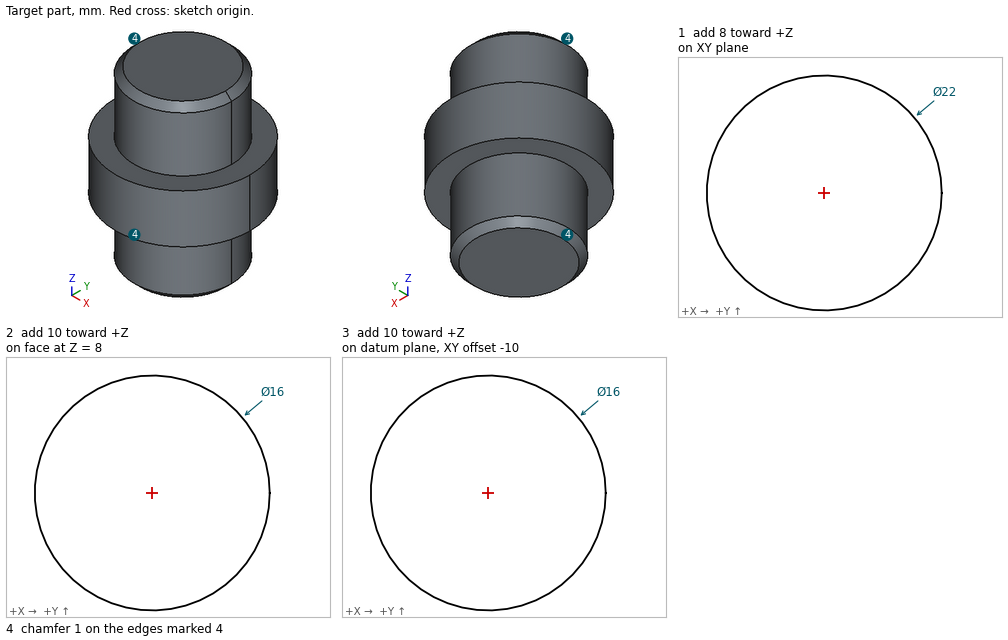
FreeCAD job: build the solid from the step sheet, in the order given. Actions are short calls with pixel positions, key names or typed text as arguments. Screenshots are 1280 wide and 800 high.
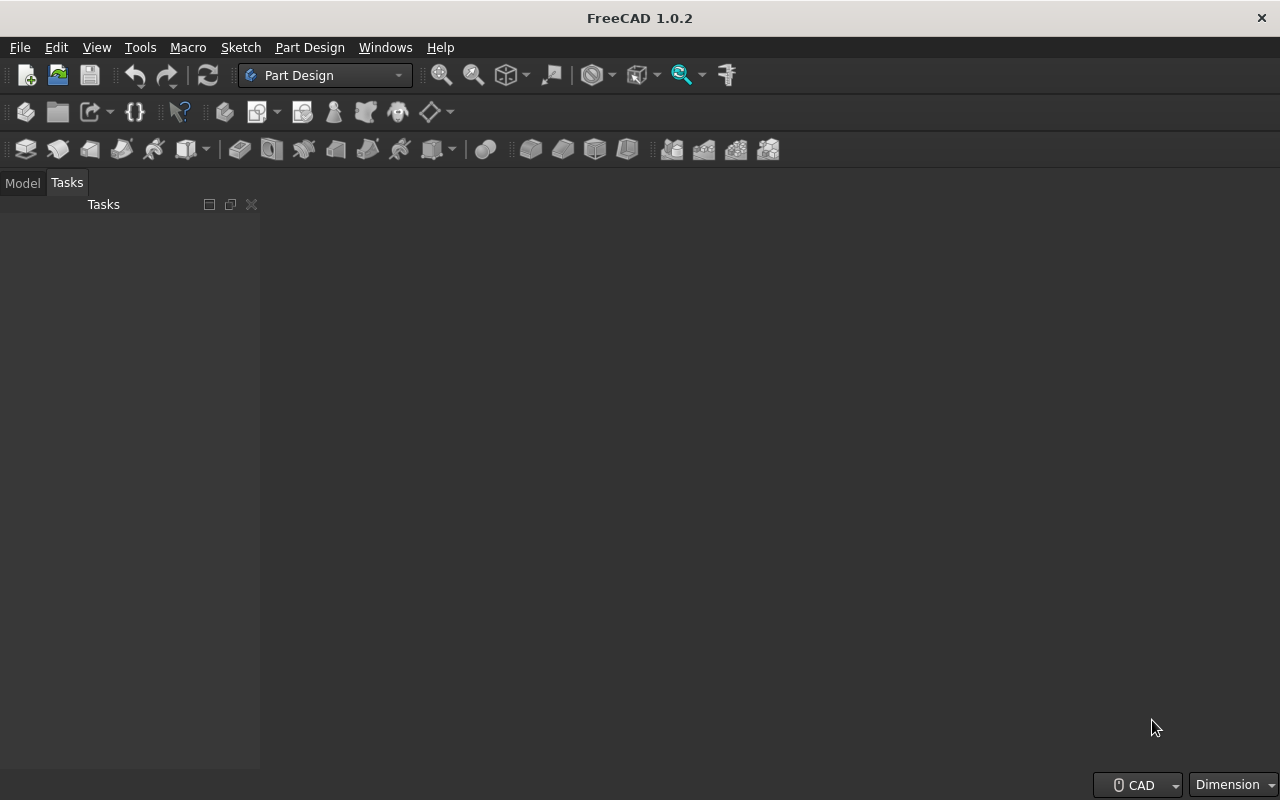
click(26, 76)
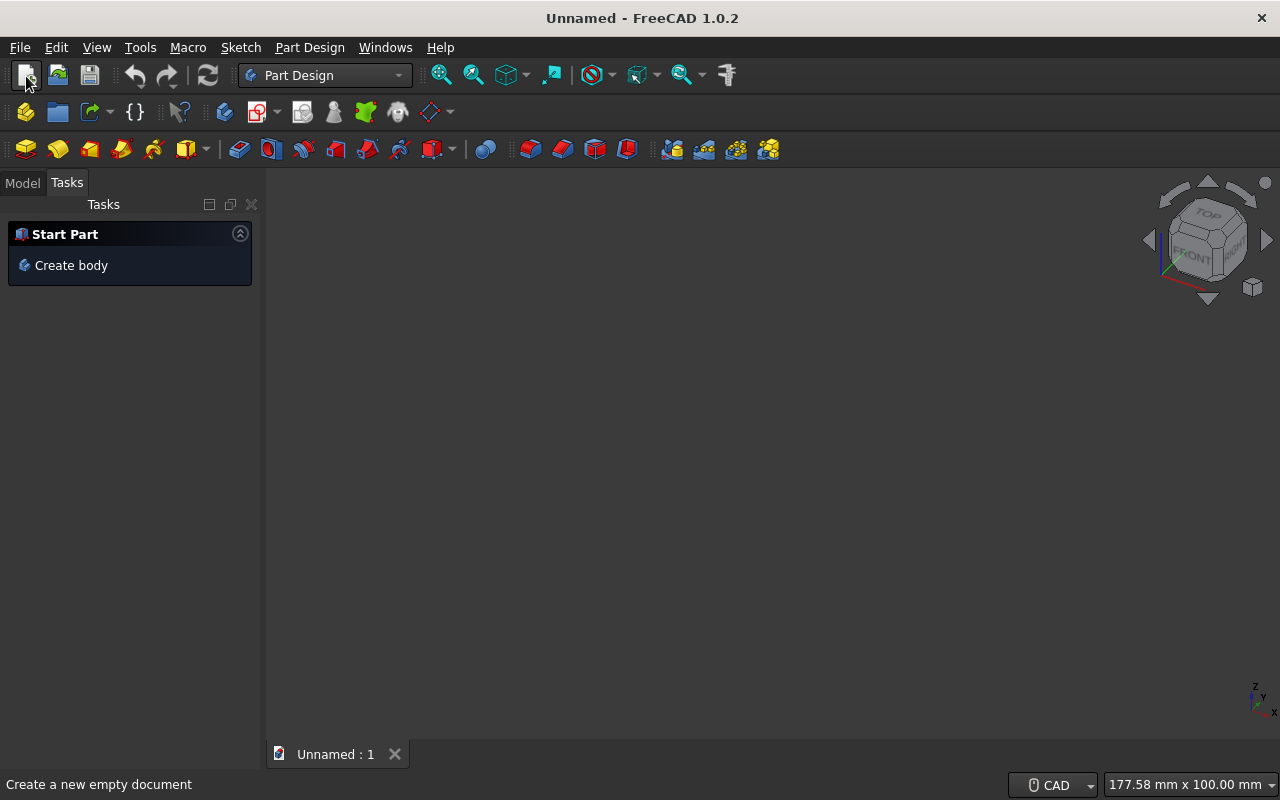
click(258, 112)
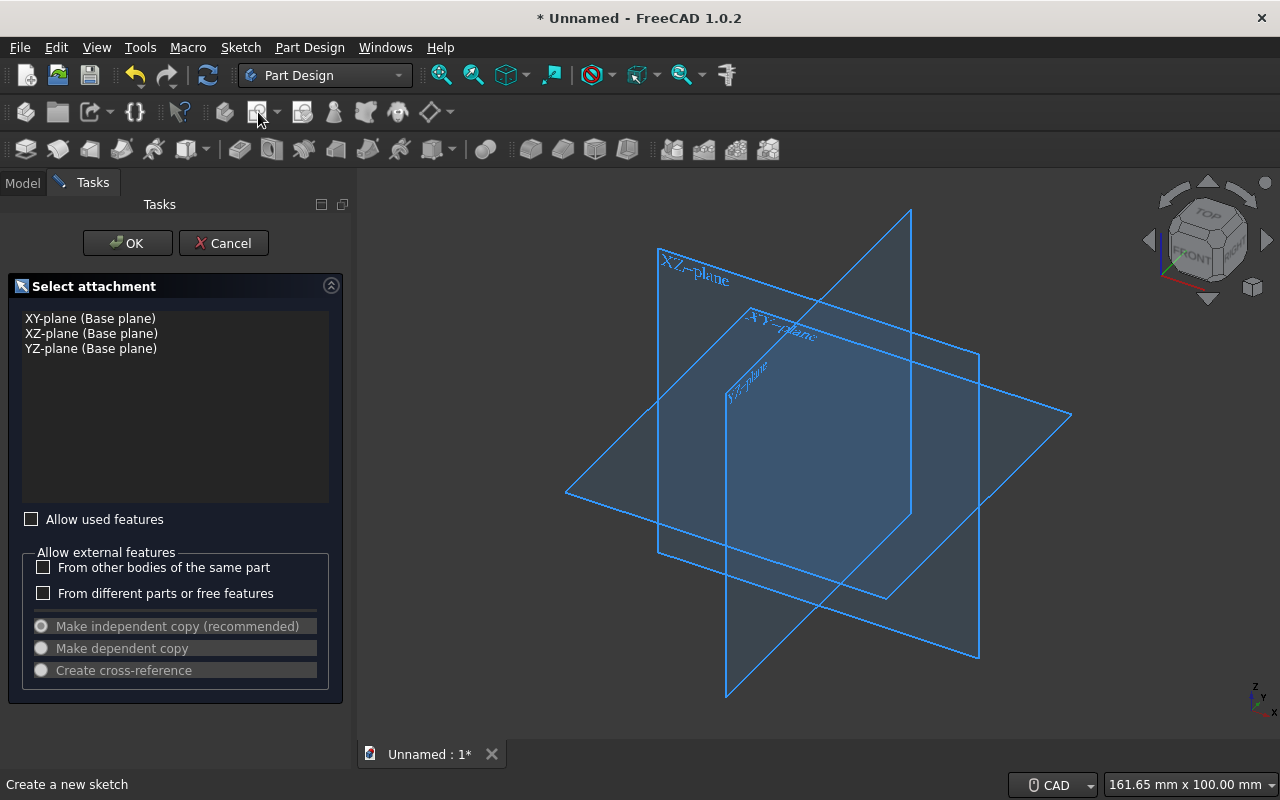
click(82, 318)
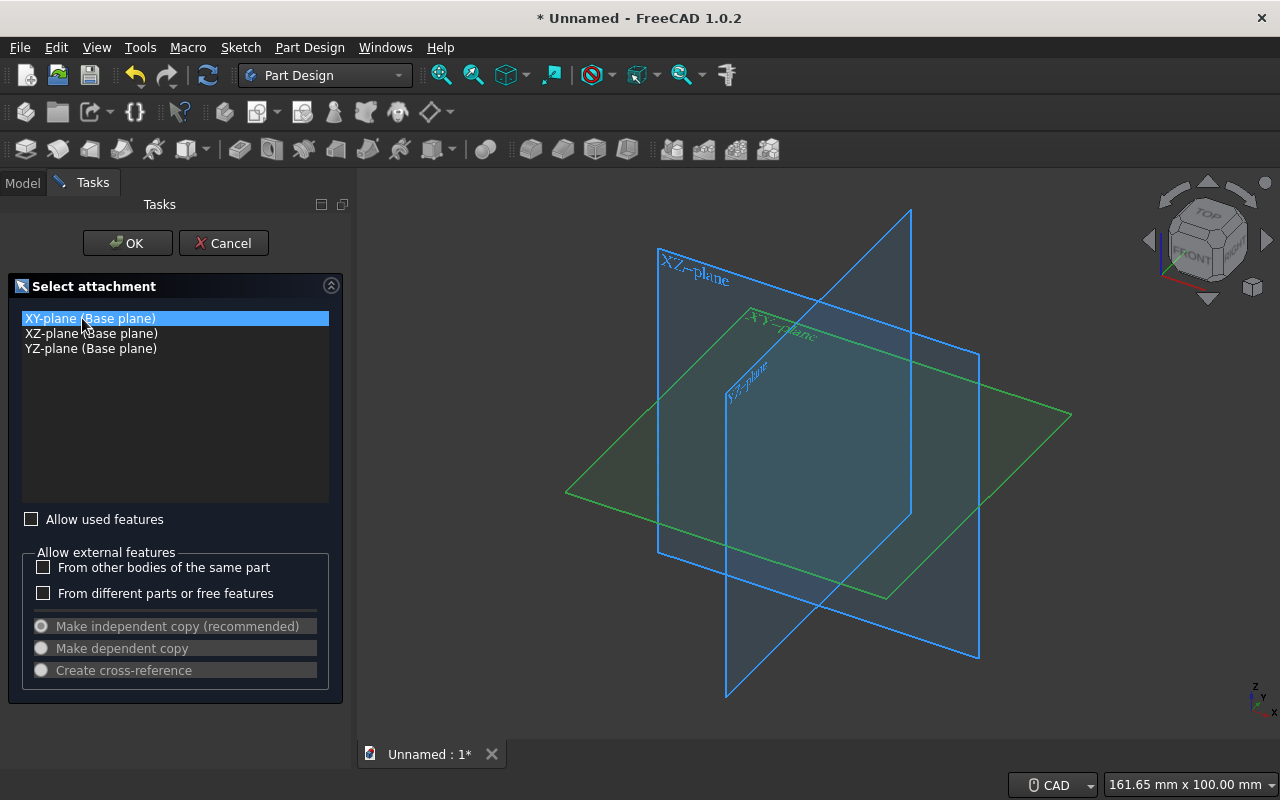
click(128, 243)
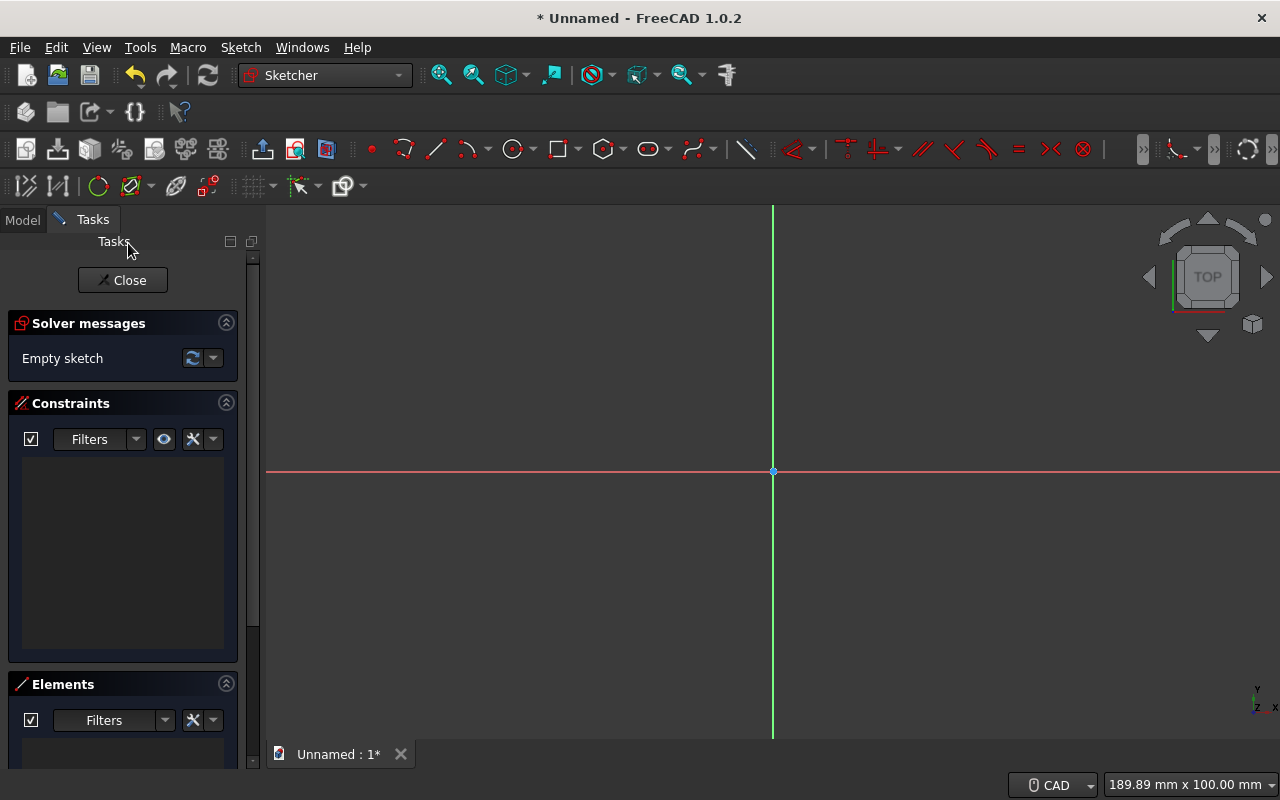
scroll(813, 472, up, 5)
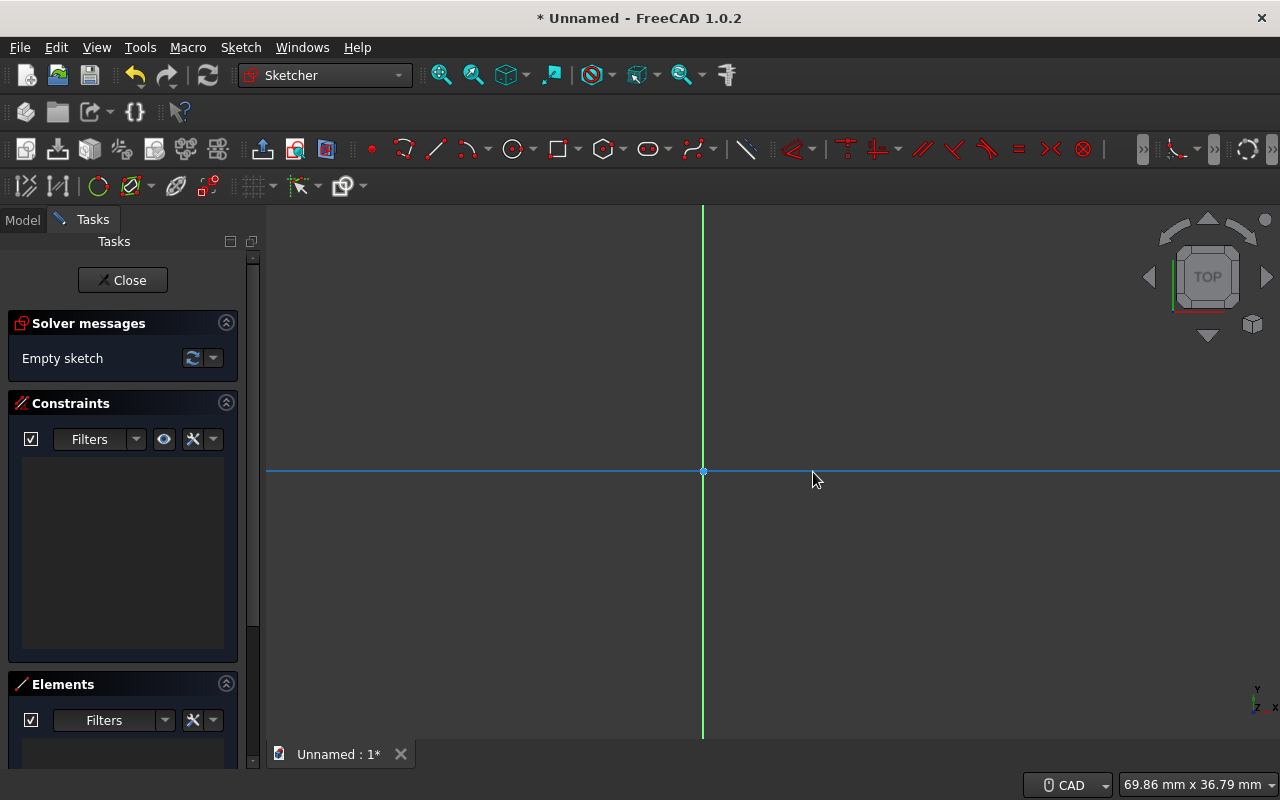
key(g)
key(c)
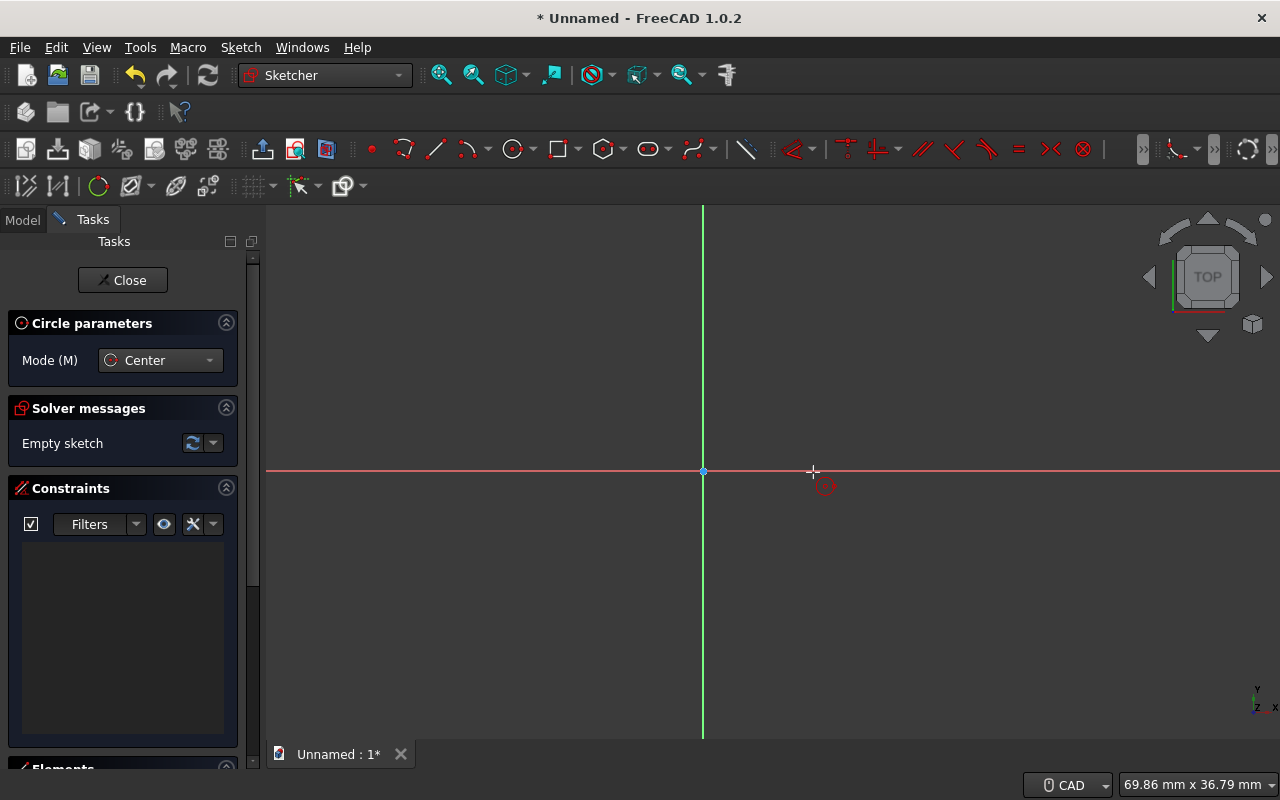
click(703, 471)
click(816, 358)
key(Escape)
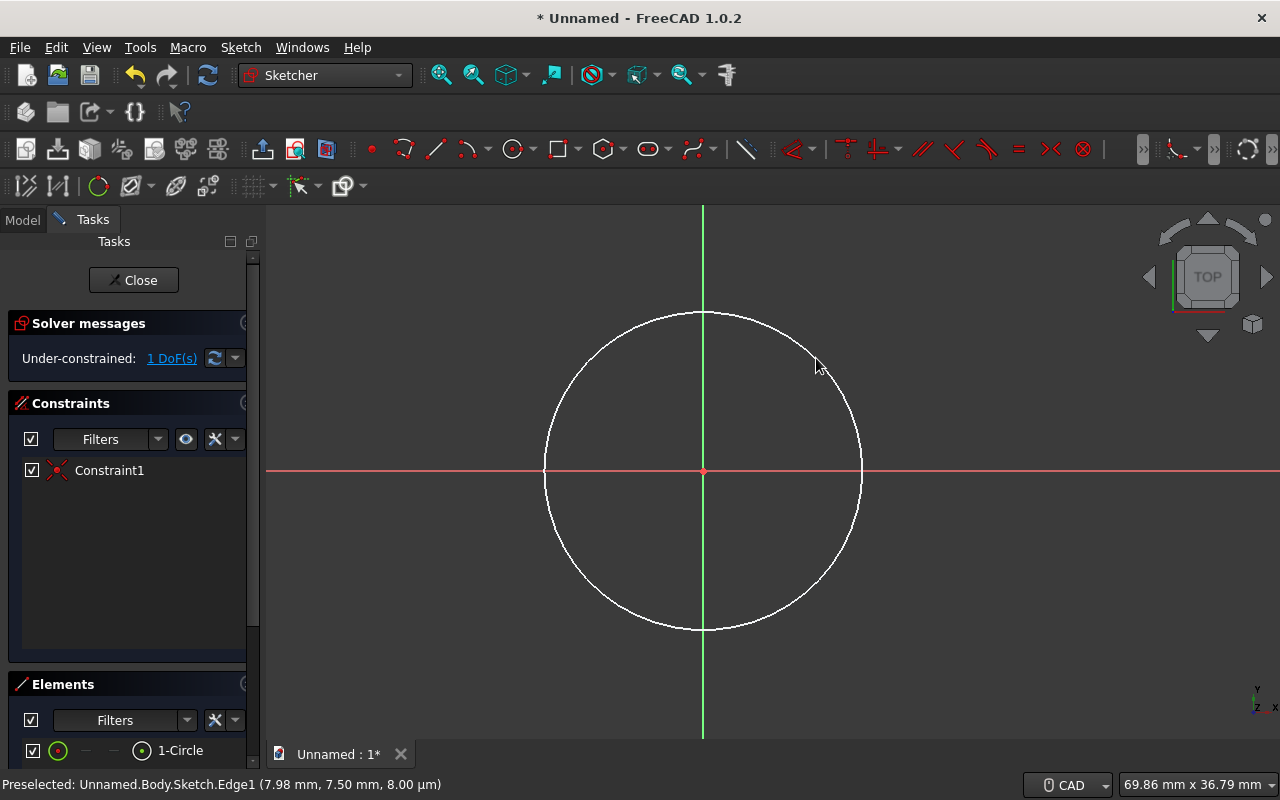
click(815, 358)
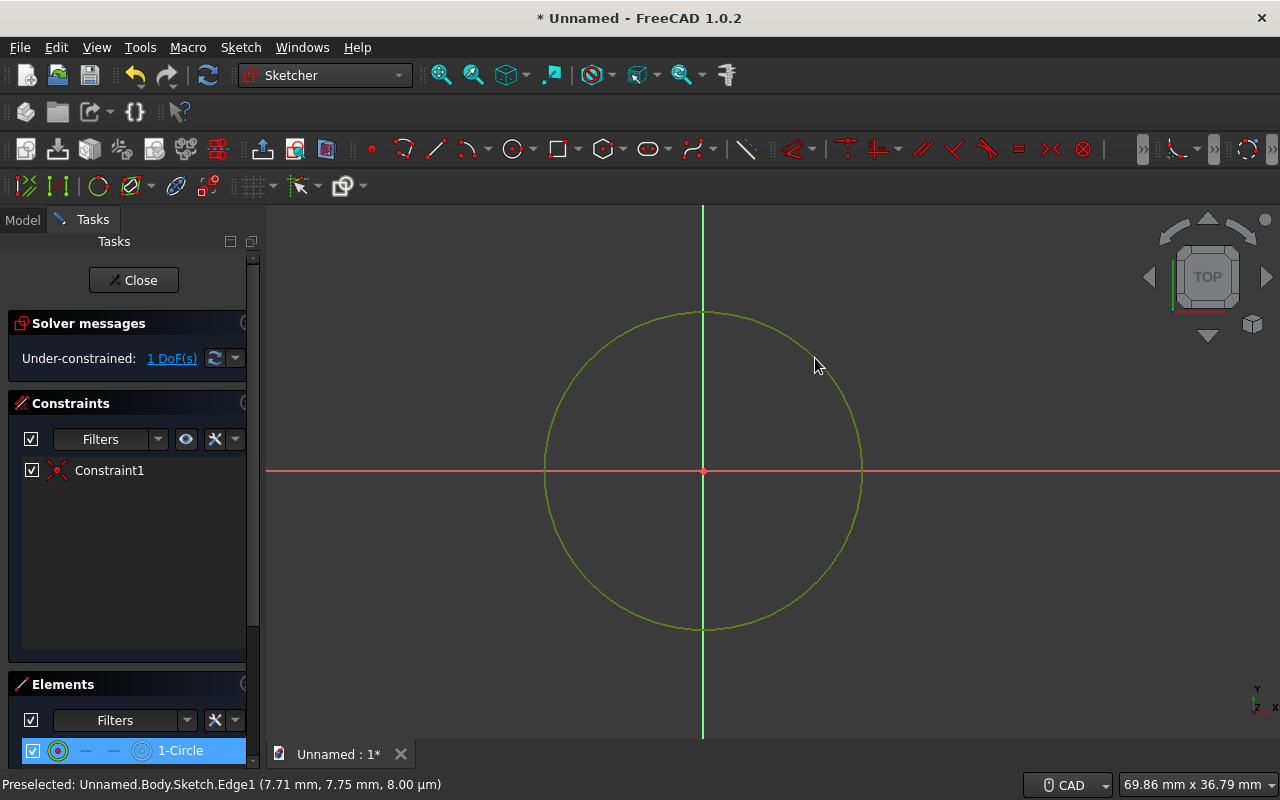
click(814, 150)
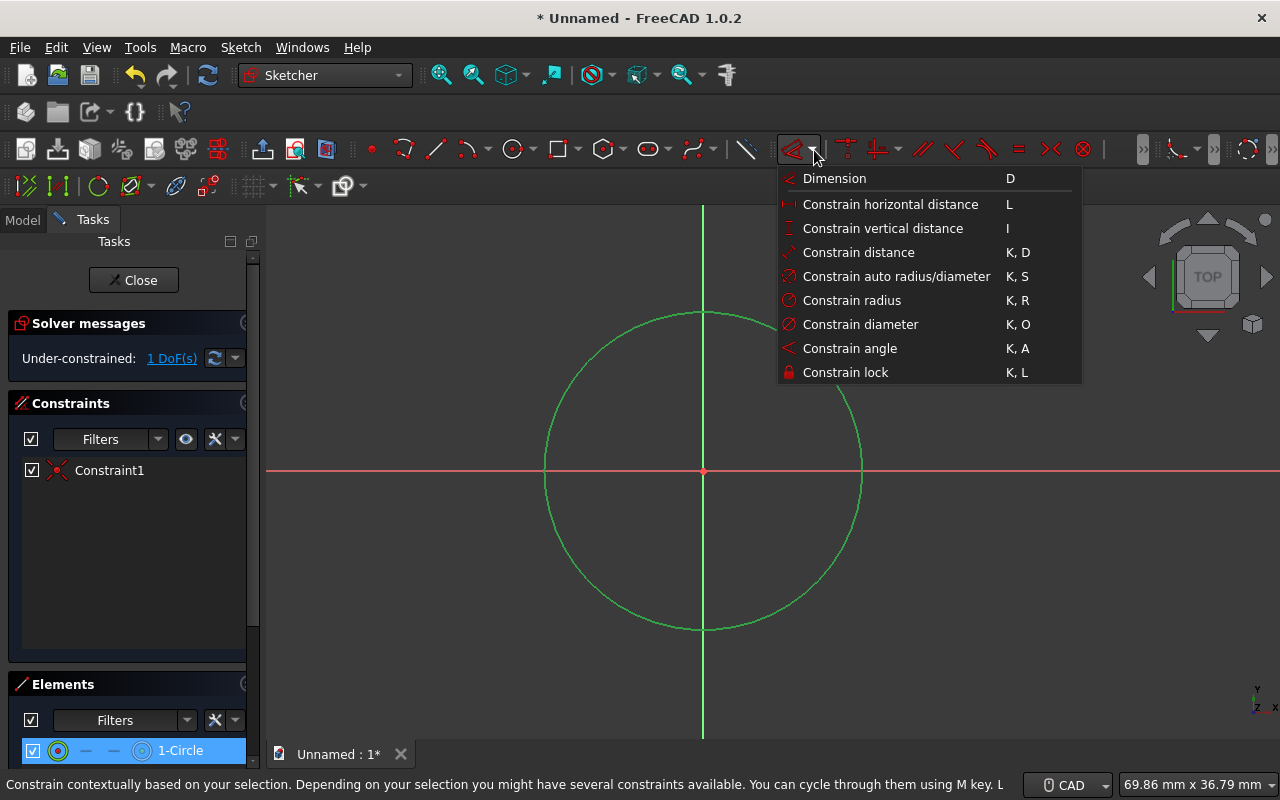
click(930, 324)